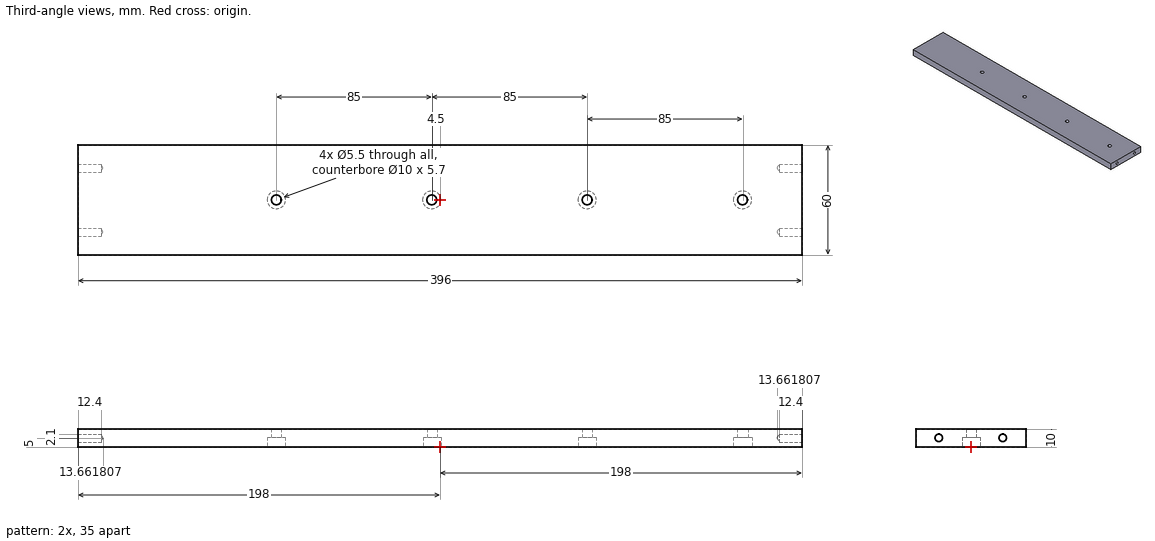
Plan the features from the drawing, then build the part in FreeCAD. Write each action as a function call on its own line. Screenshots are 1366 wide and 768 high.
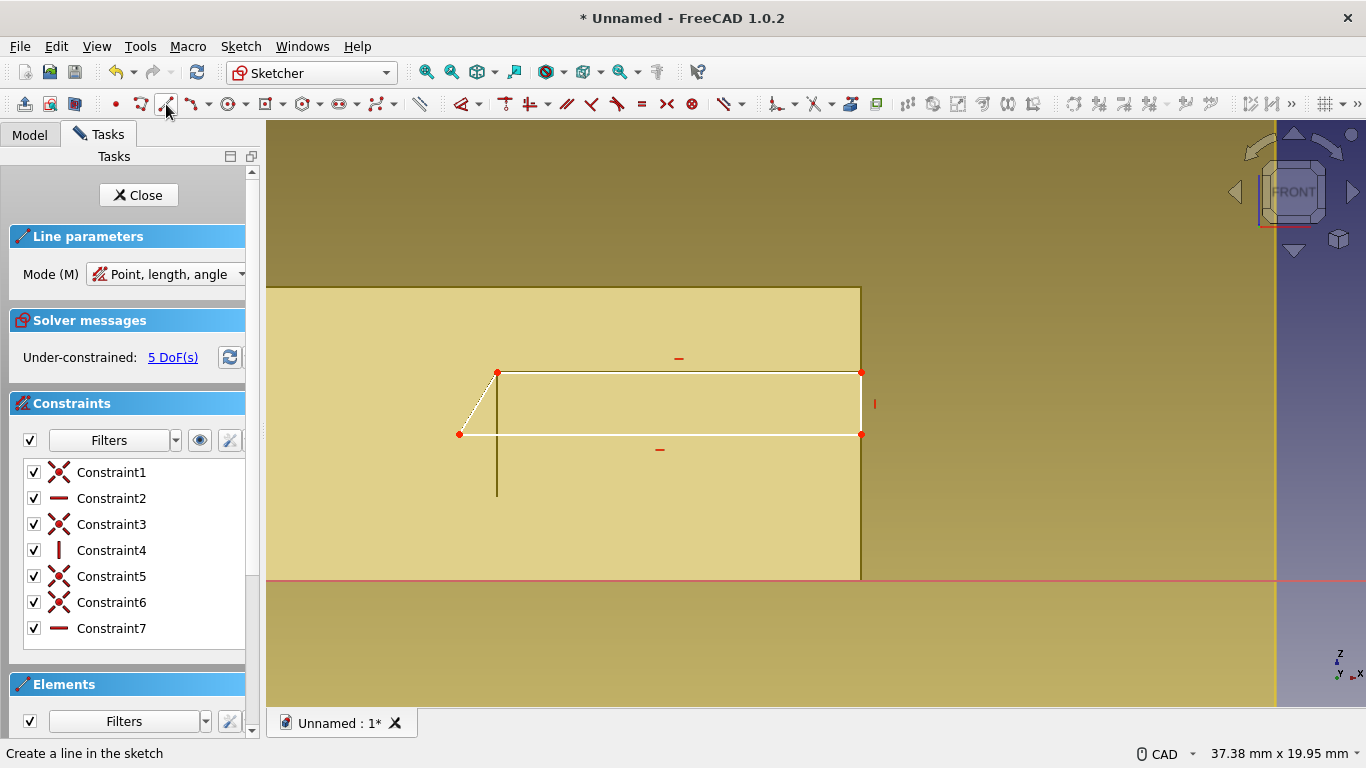
click(902, 434)
click(1022, 434)
key(Escape)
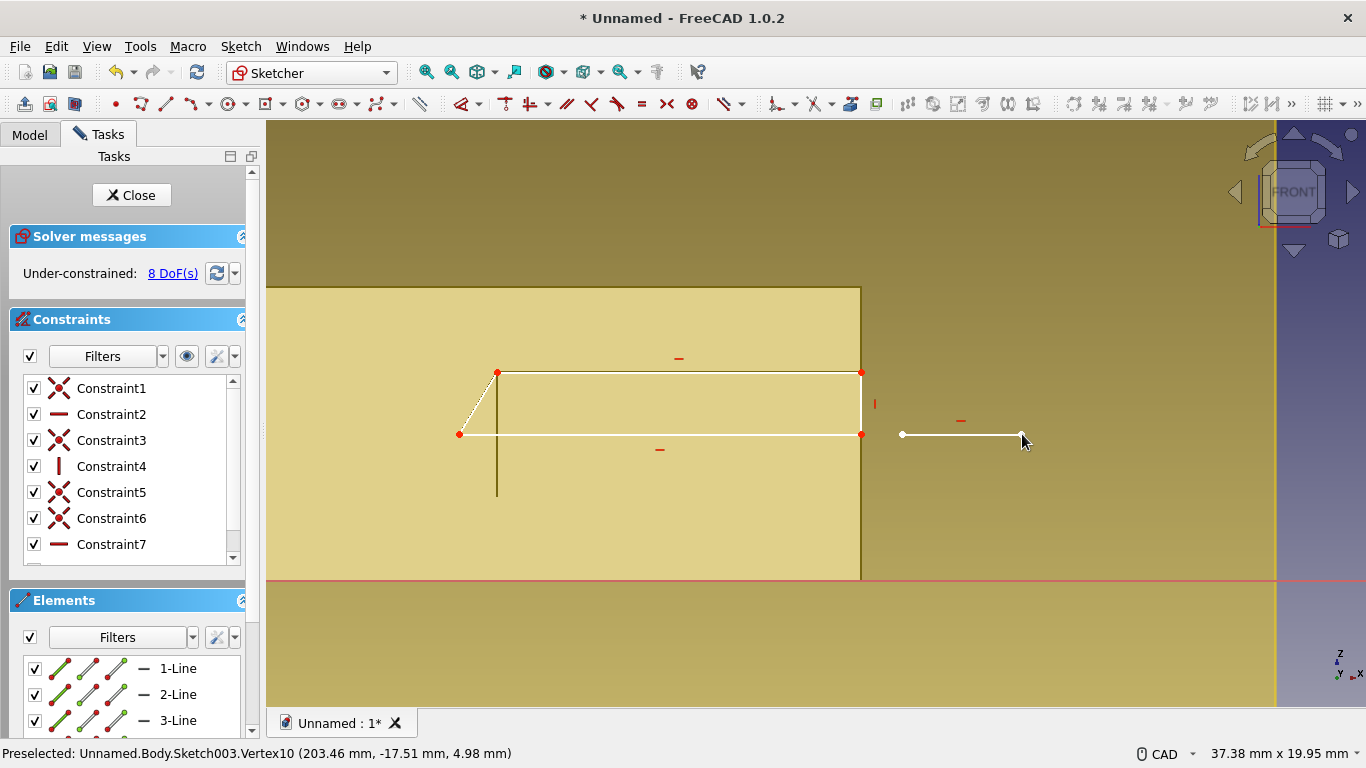
click(938, 435)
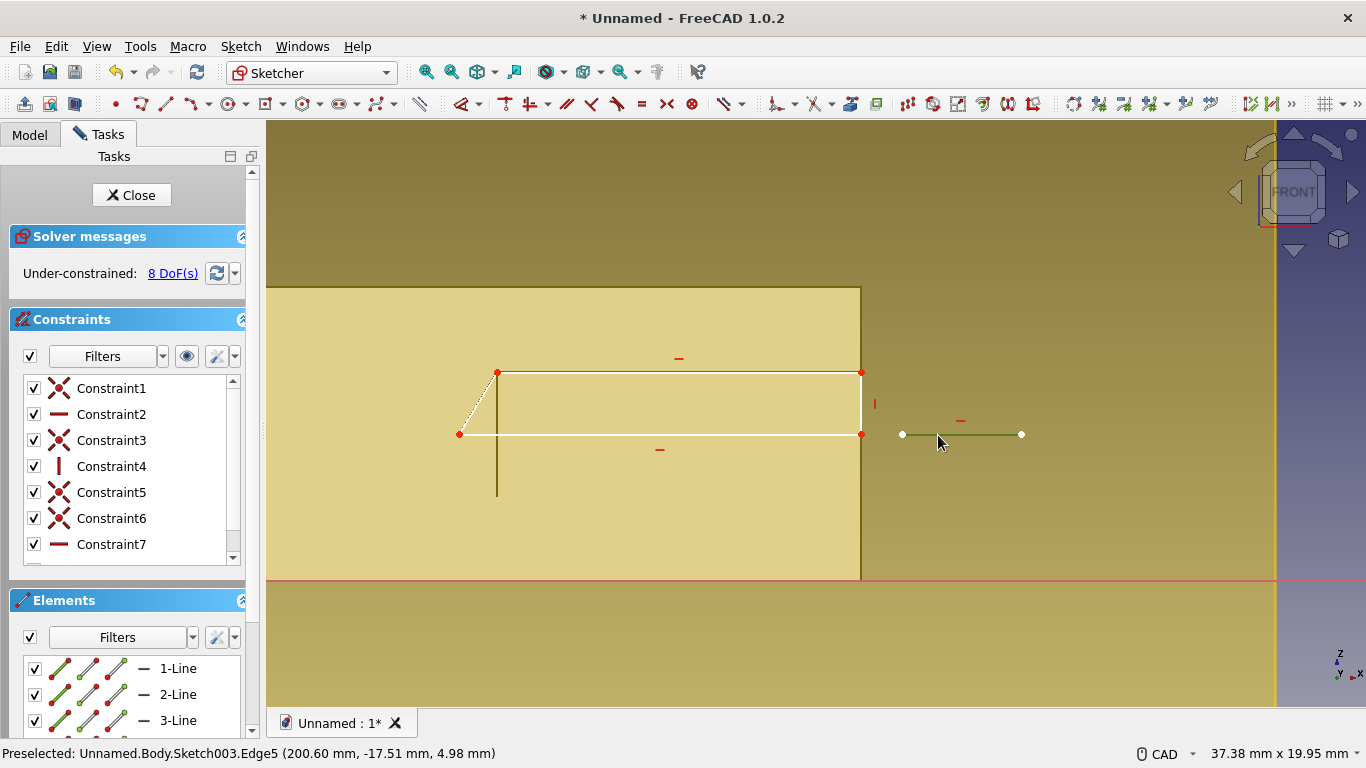
key(g)
key(n)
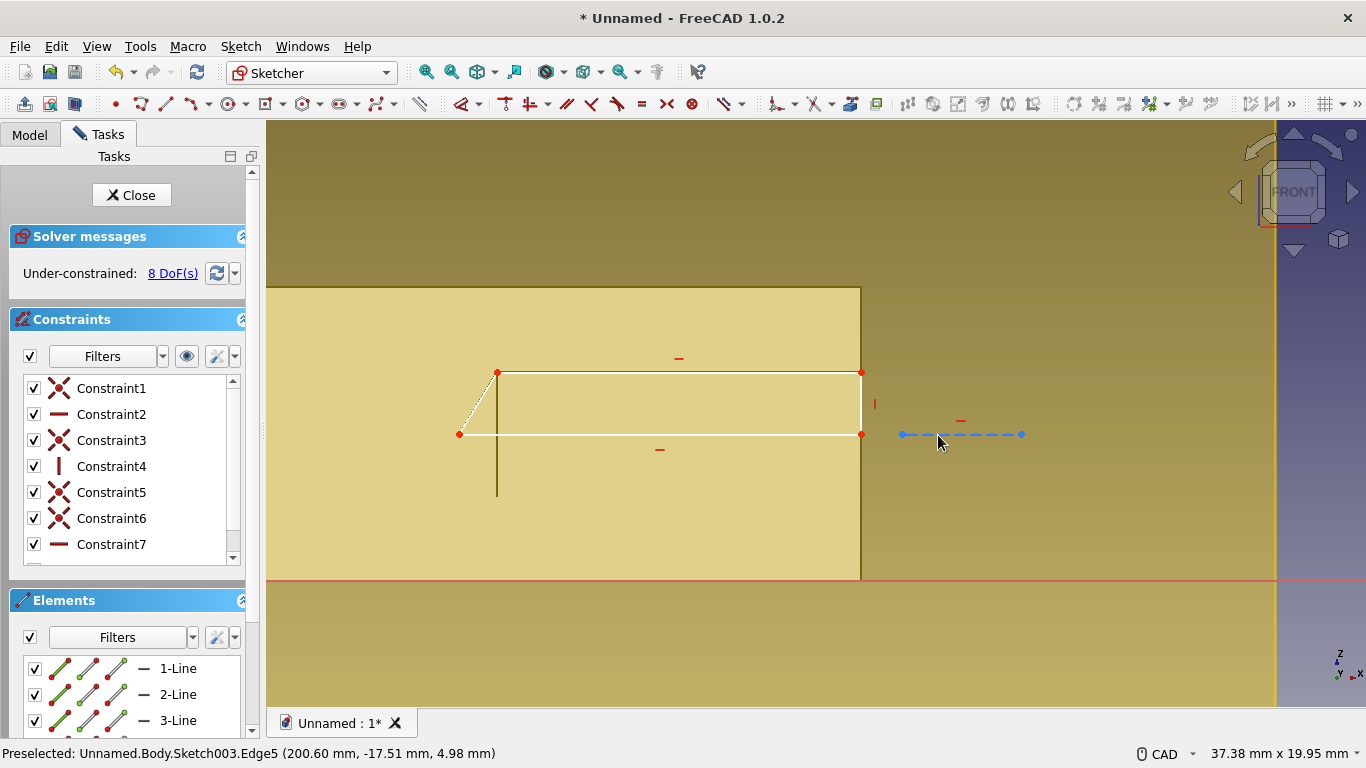
click(460, 104)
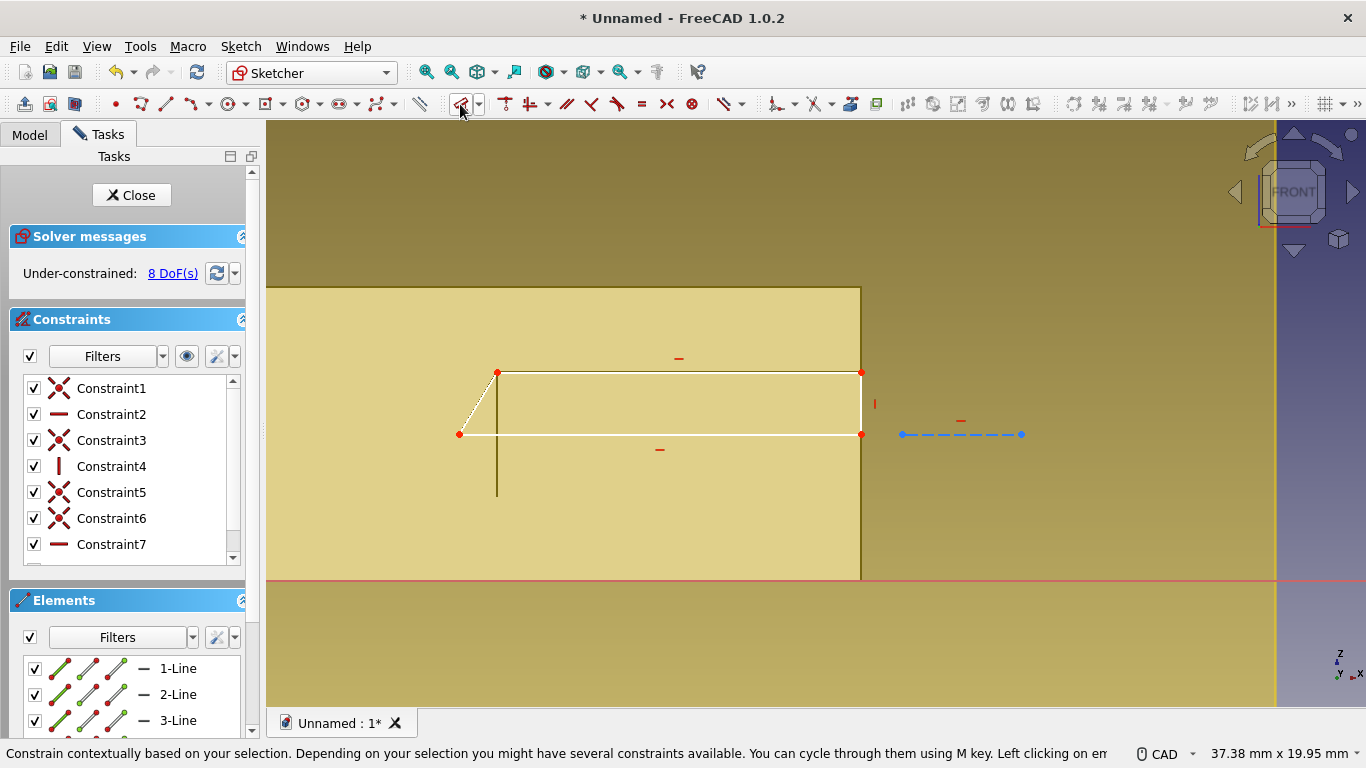
click(459, 435)
click(493, 508)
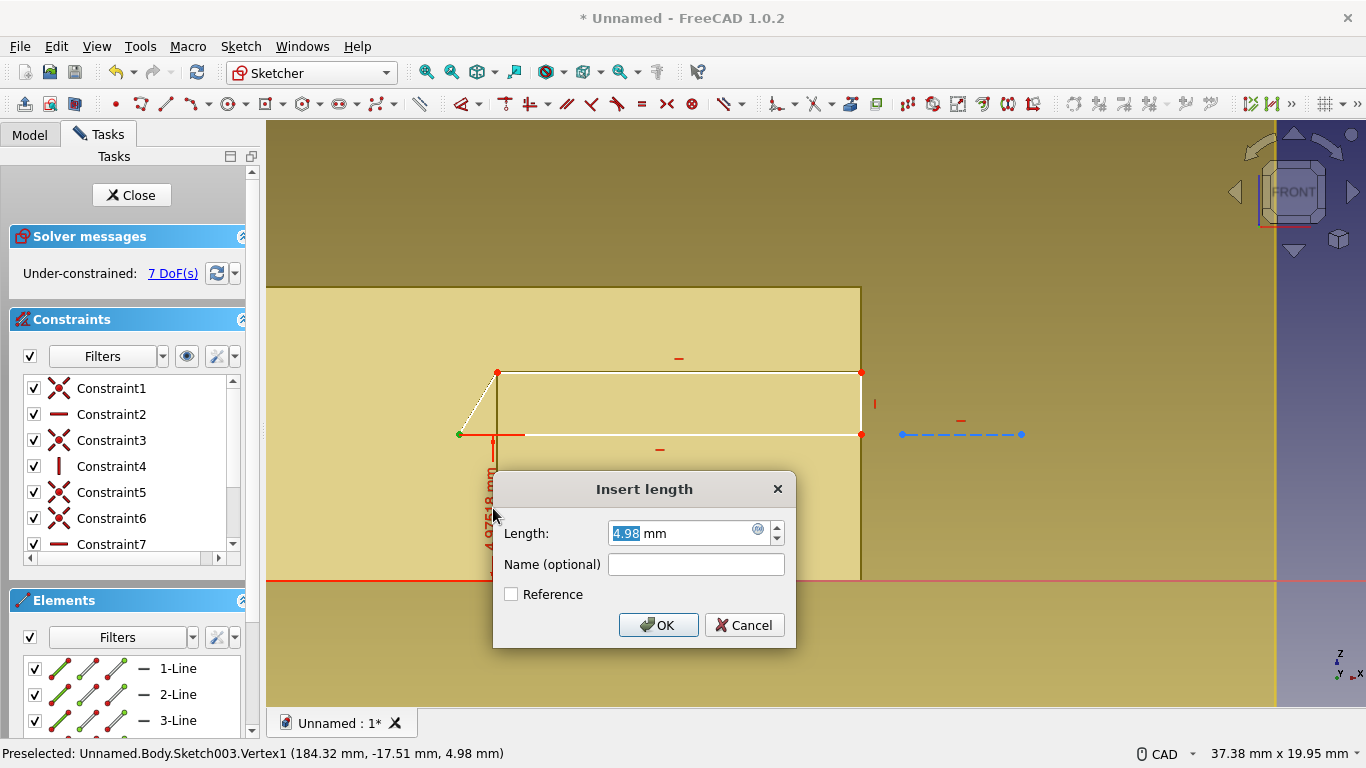
text(5)
key(Return)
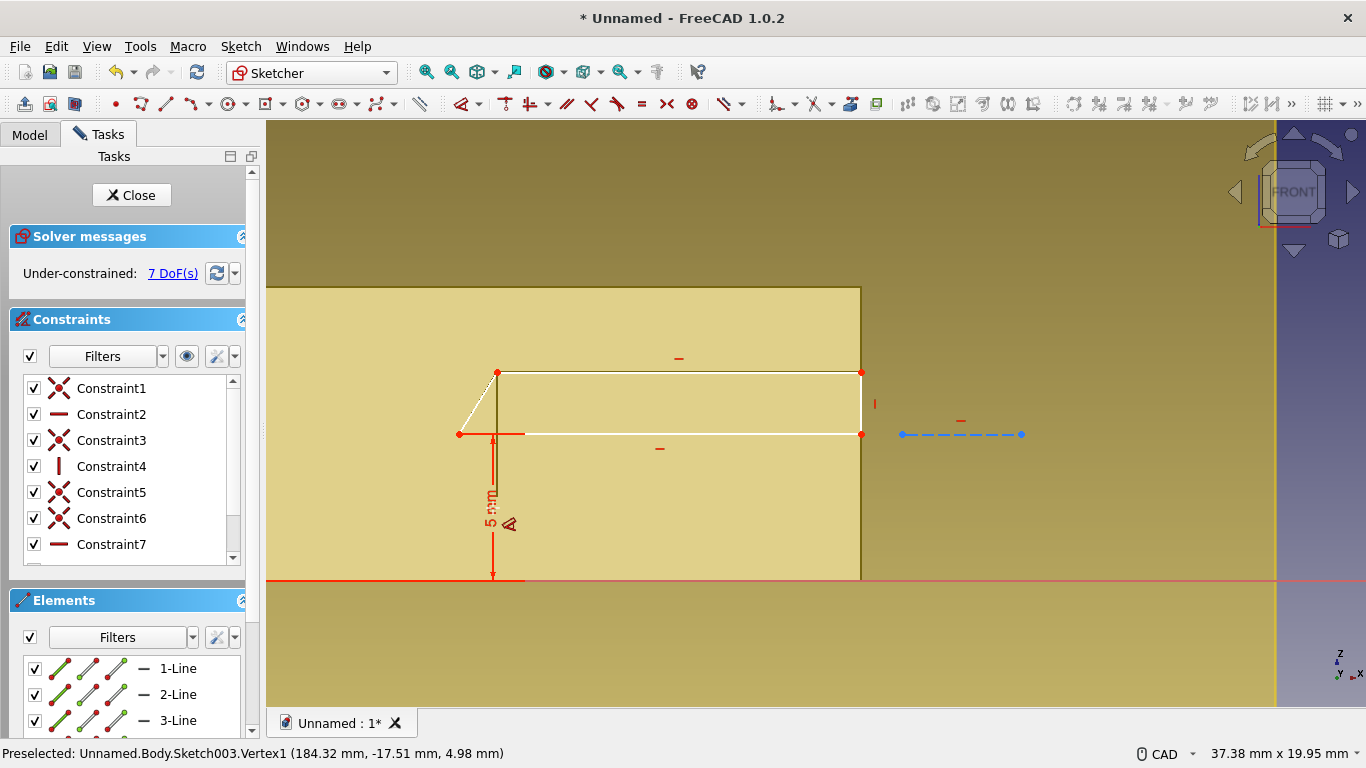
click(902, 435)
click(936, 508)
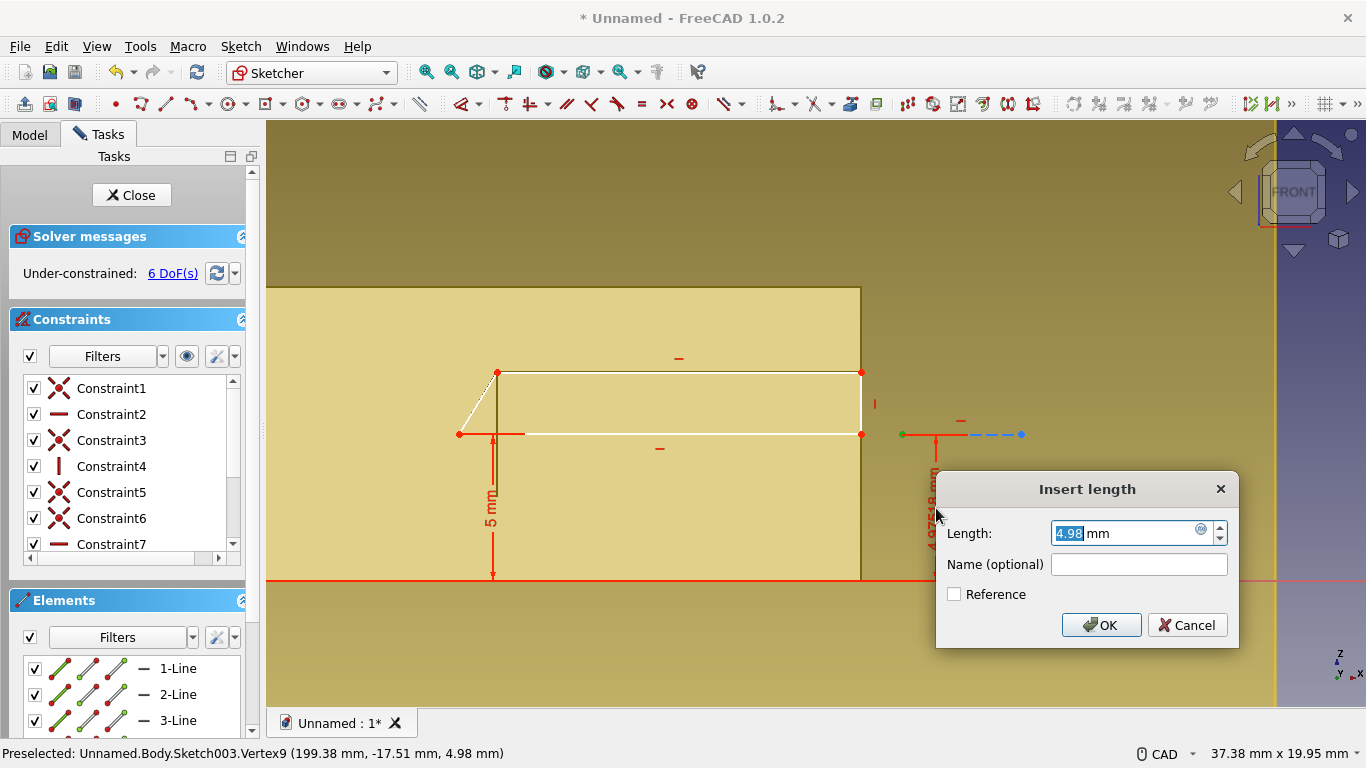
text(5)
key(Return)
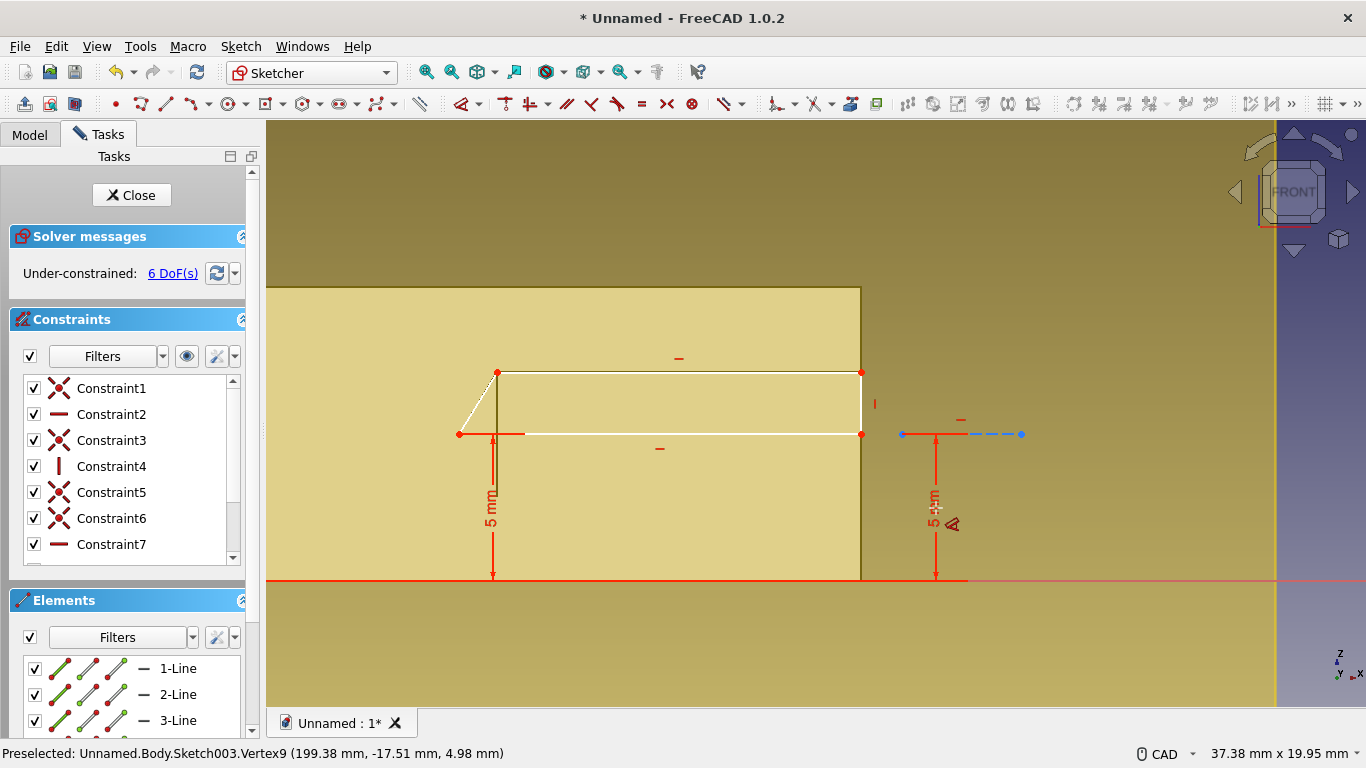
click(861, 391)
click(895, 404)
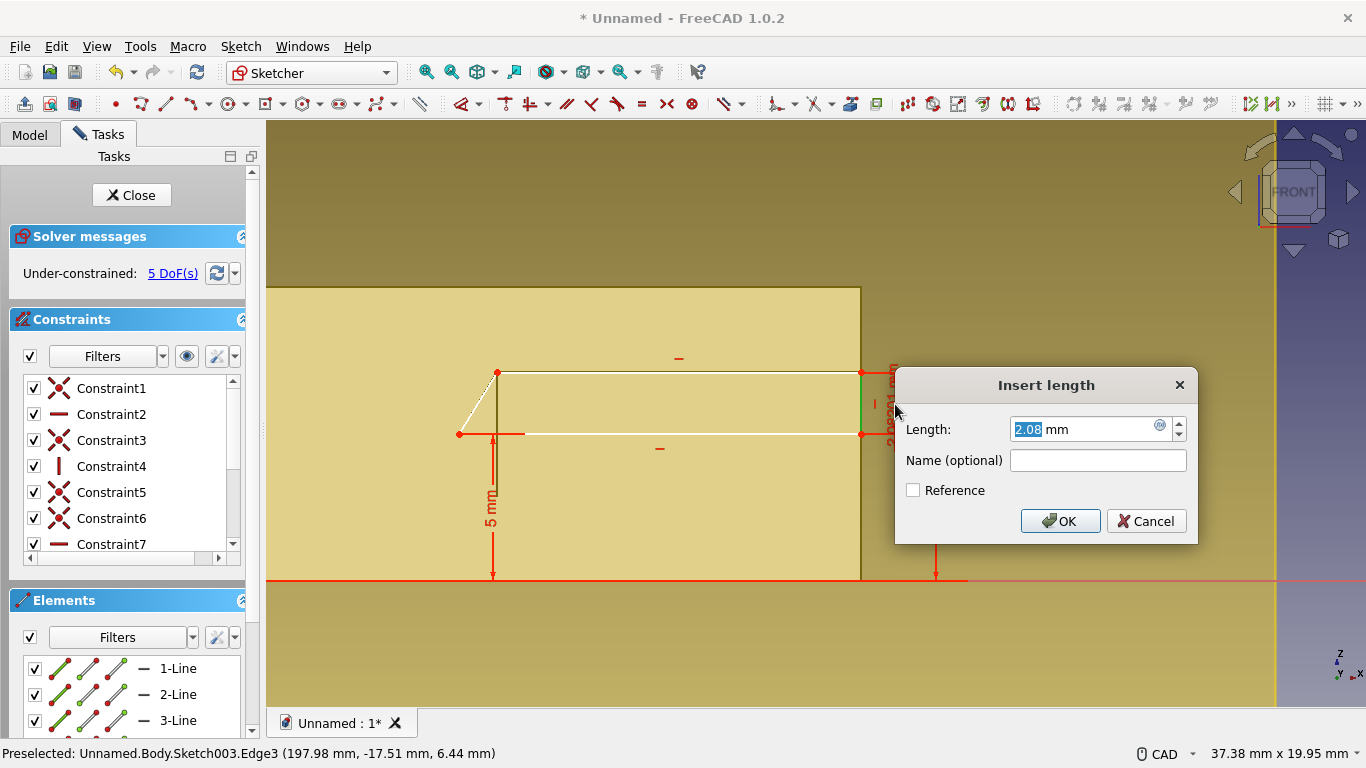
text(2.1)
key(Return)